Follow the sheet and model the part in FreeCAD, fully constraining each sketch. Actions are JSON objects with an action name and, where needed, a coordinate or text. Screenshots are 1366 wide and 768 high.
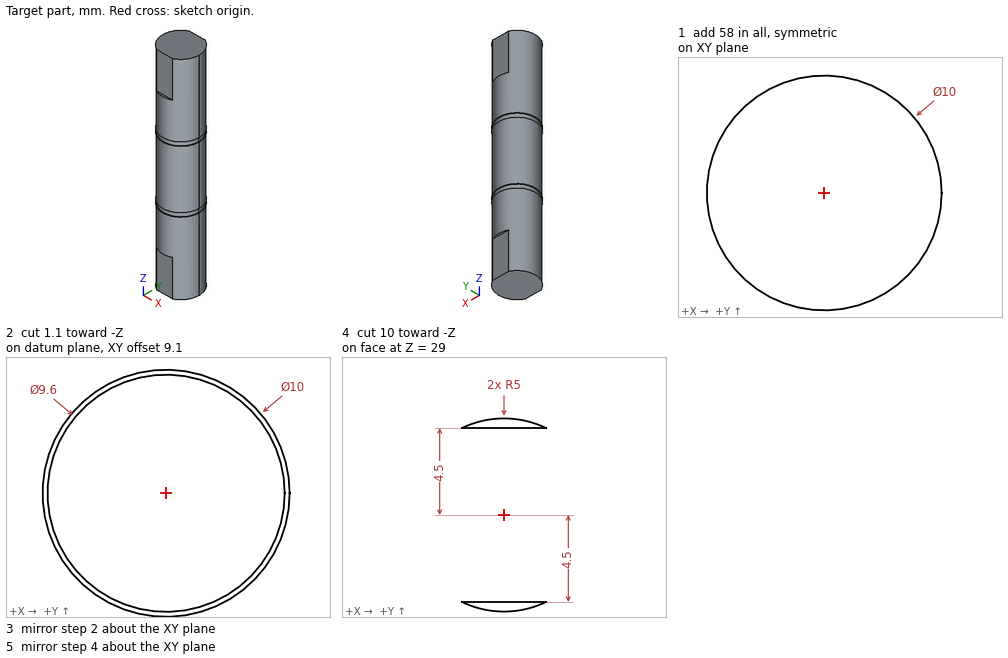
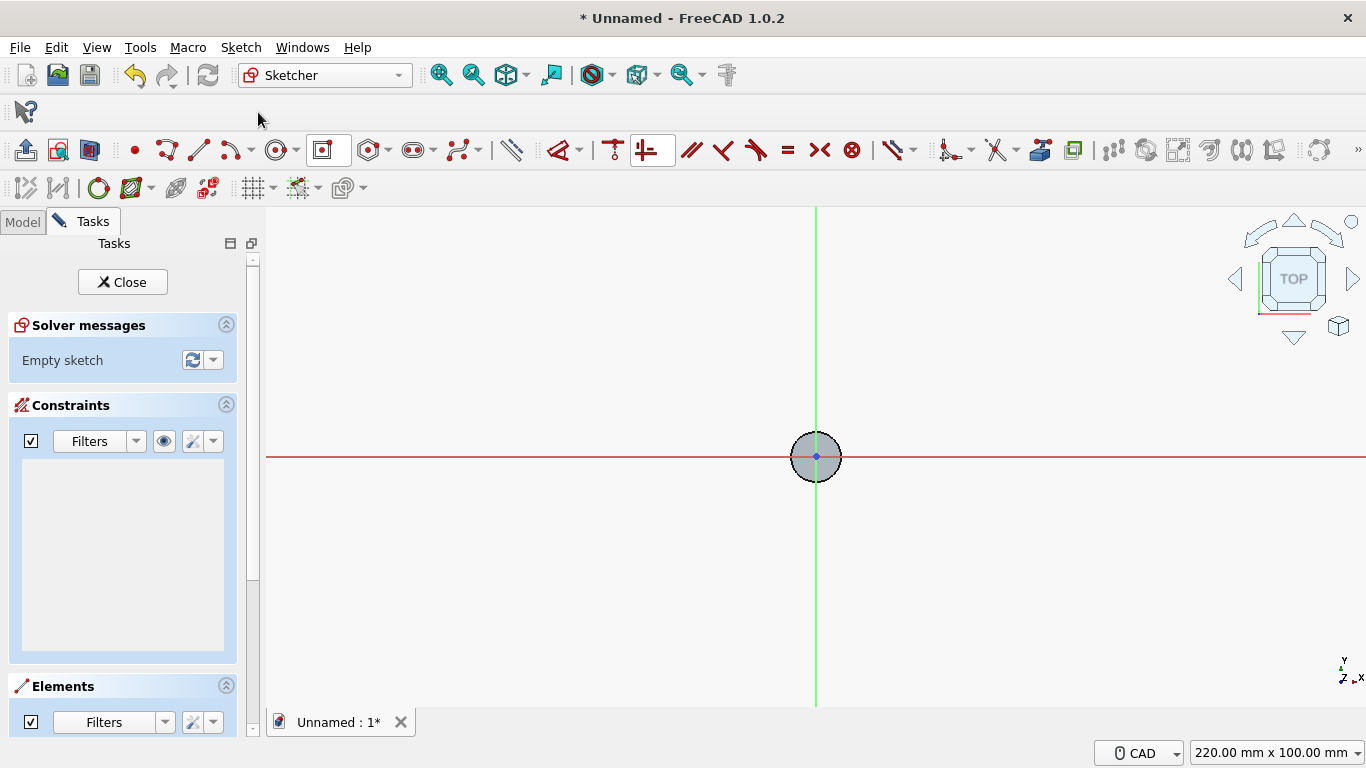
{"action": "scroll", "coordinate": [830, 457], "scroll_direction": "up", "scroll_amount": 9}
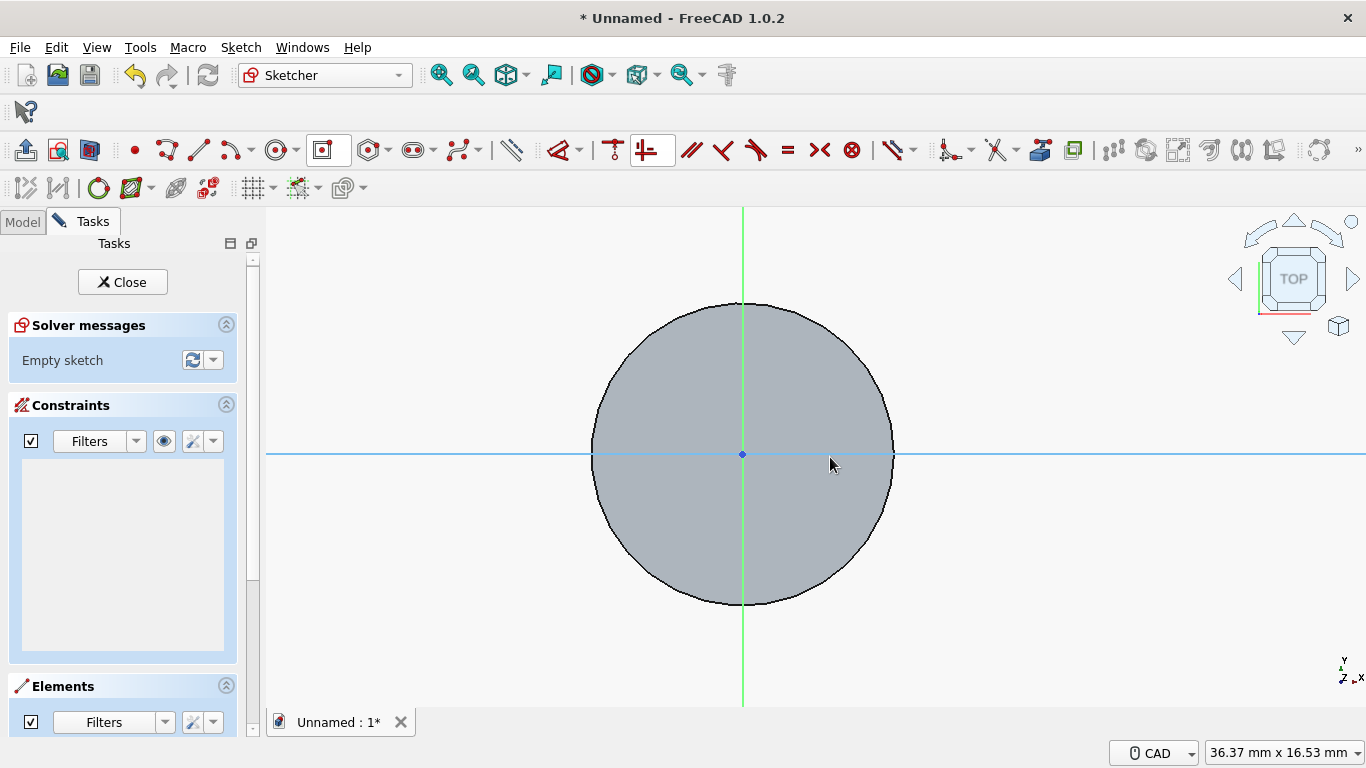
{"action": "left_click", "coordinate": [200, 150]}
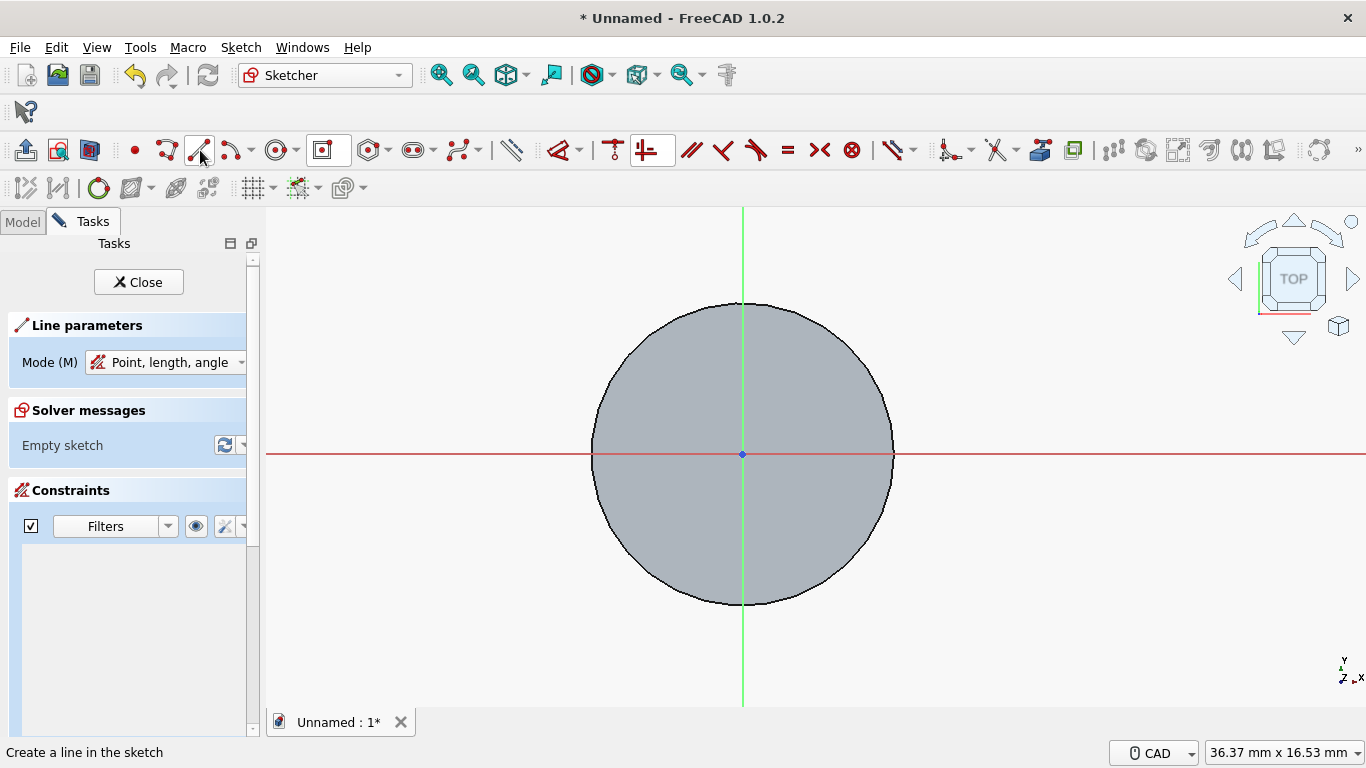
{"action": "left_click", "coordinate": [677, 318]}
{"action": "left_click", "coordinate": [809, 318]}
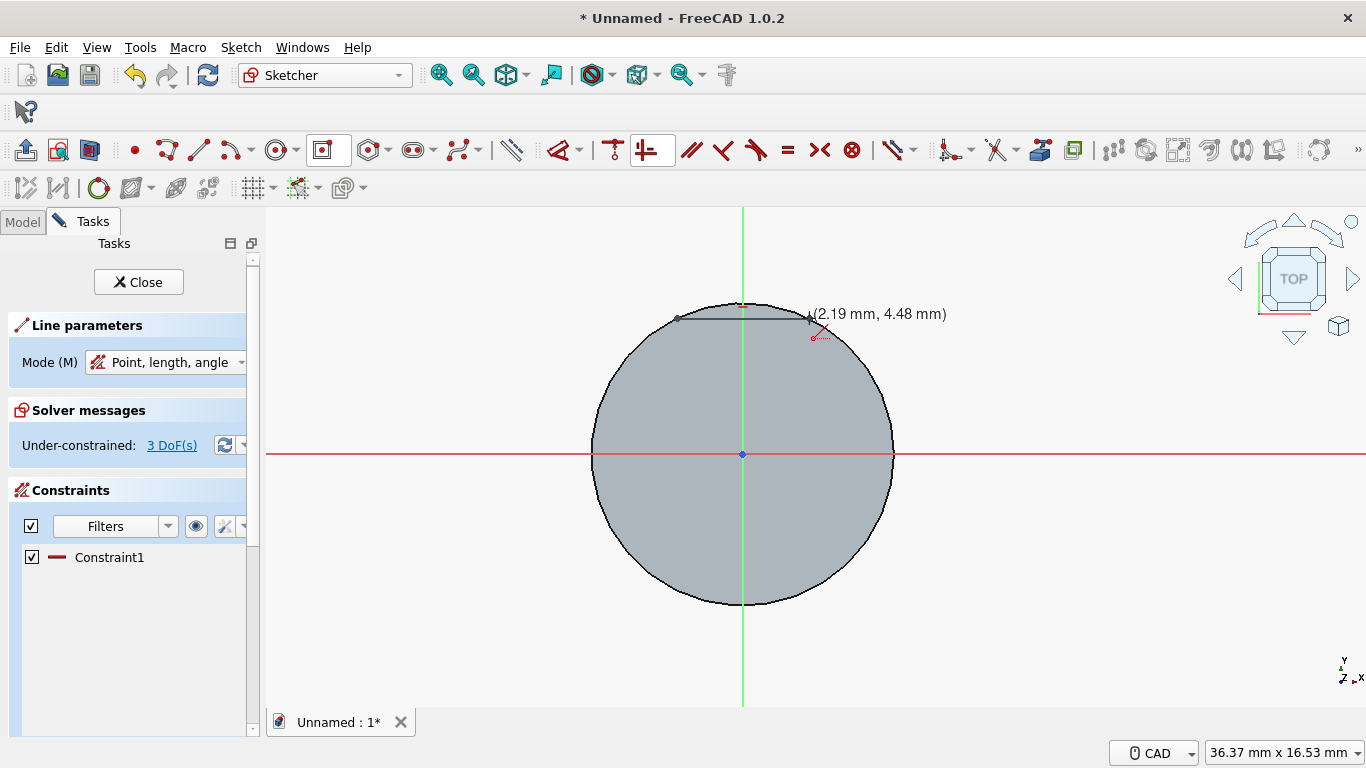
{"action": "left_click", "coordinate": [254, 150]}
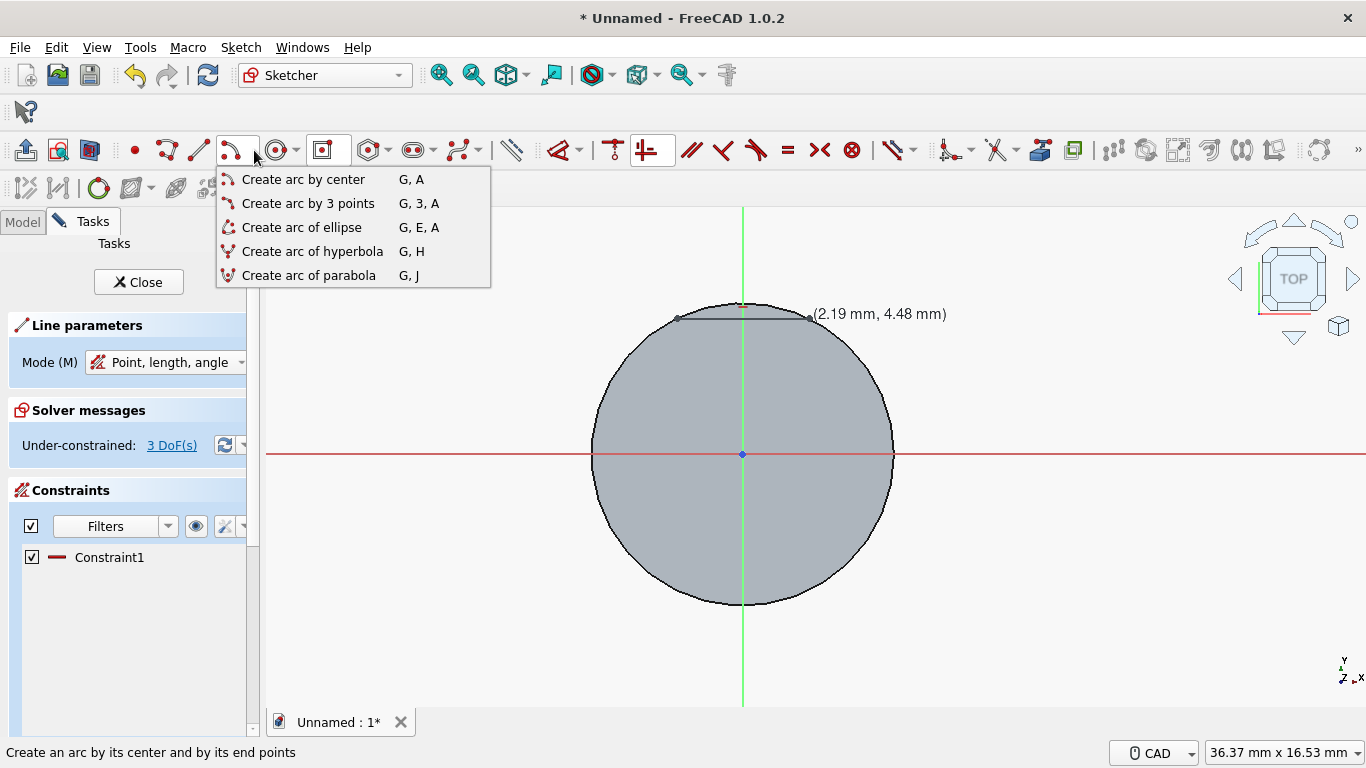
{"action": "left_click", "coordinate": [354, 203]}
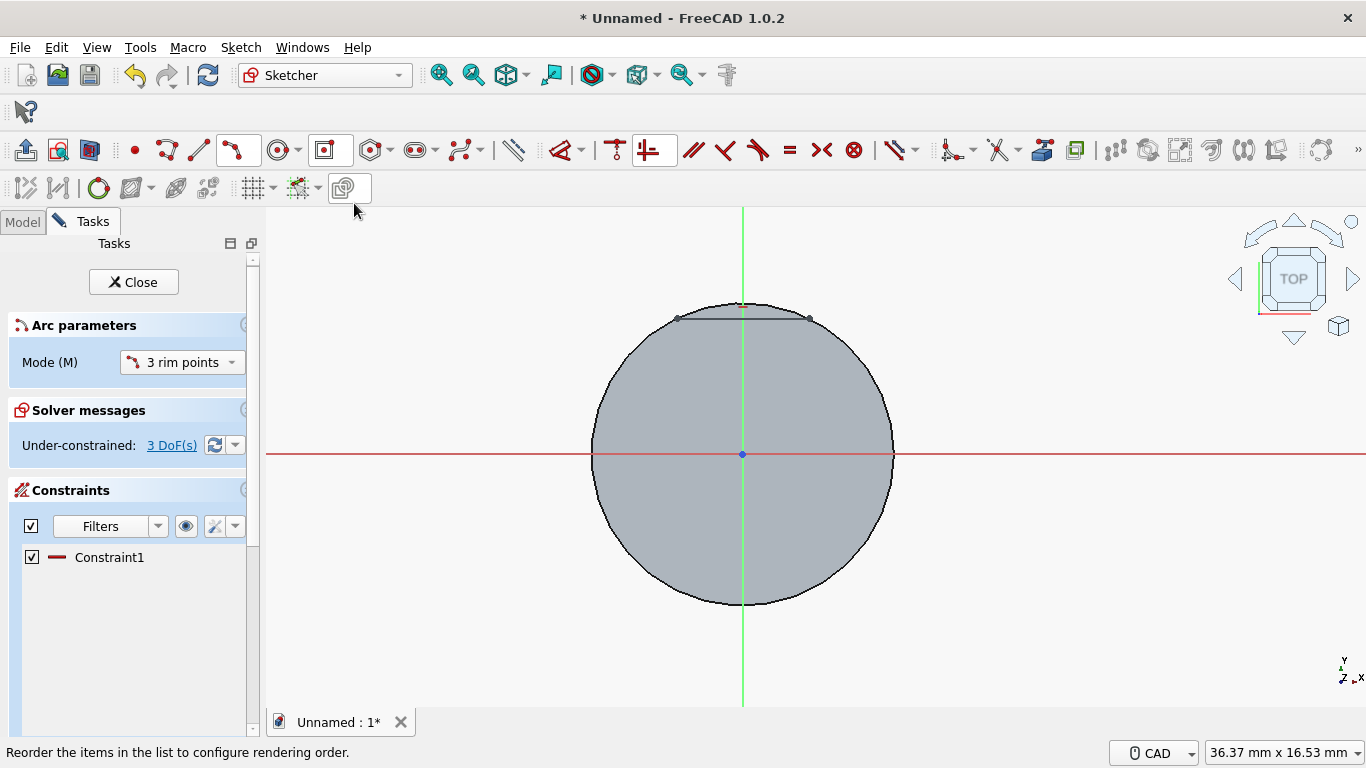
{"action": "left_click", "coordinate": [809, 319]}
{"action": "left_click", "coordinate": [677, 319]}
{"action": "left_click", "coordinate": [756, 304]}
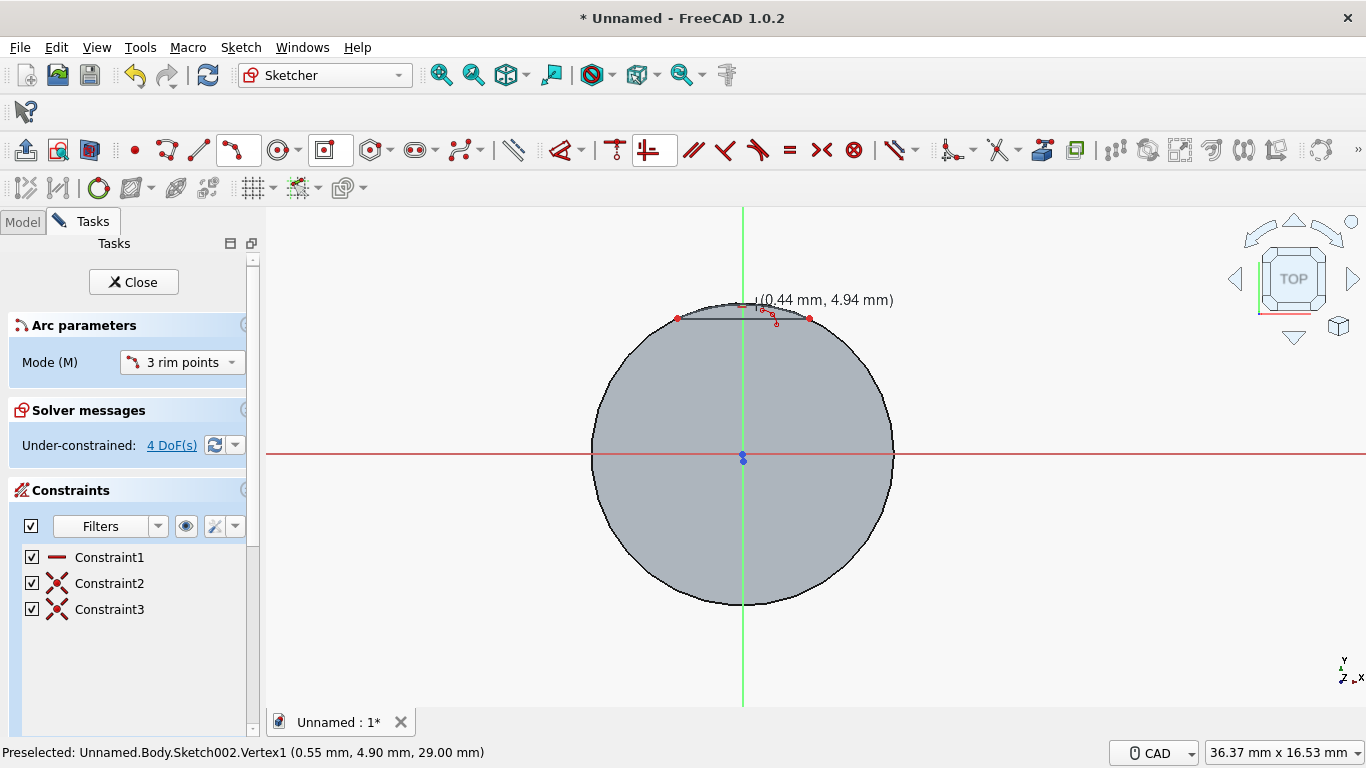
{"action": "key", "text": "g l"}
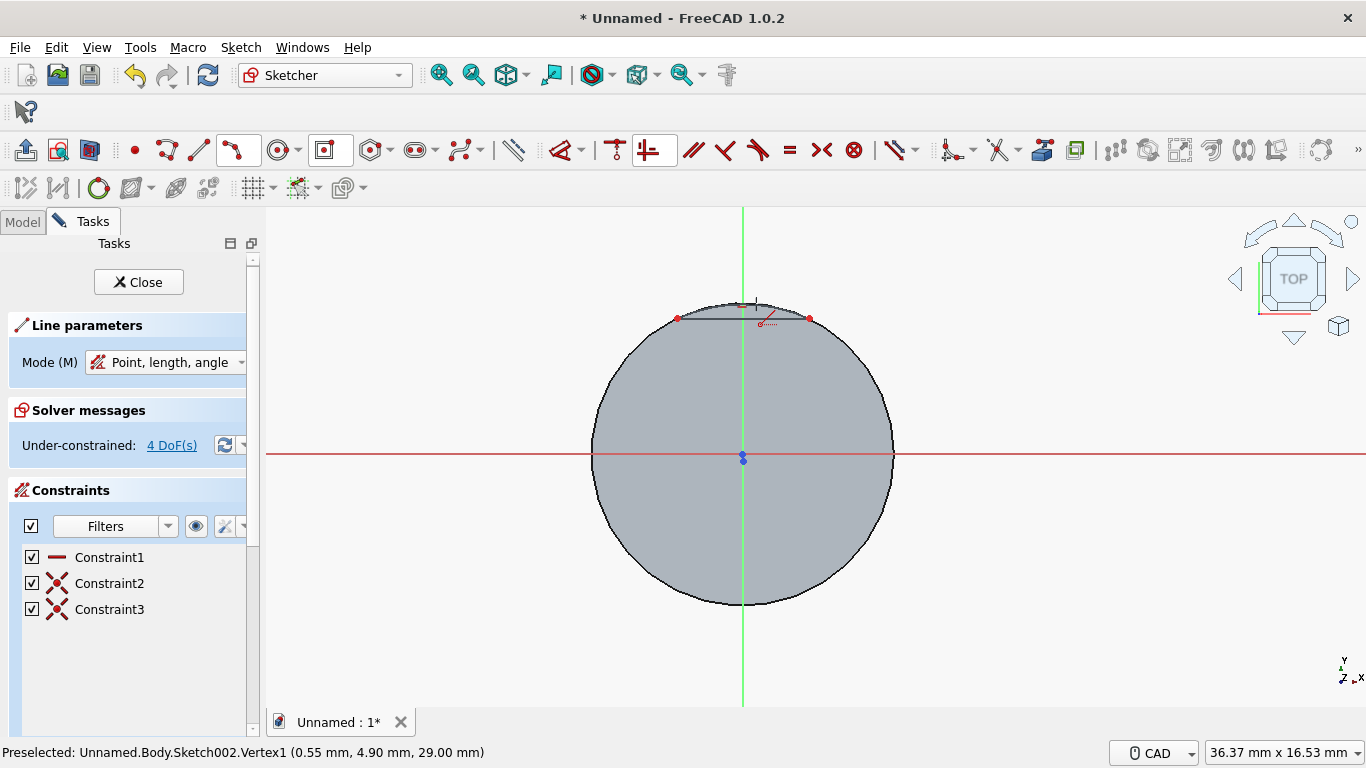
{"action": "left_click", "coordinate": [809, 591]}
{"action": "left_click", "coordinate": [677, 591]}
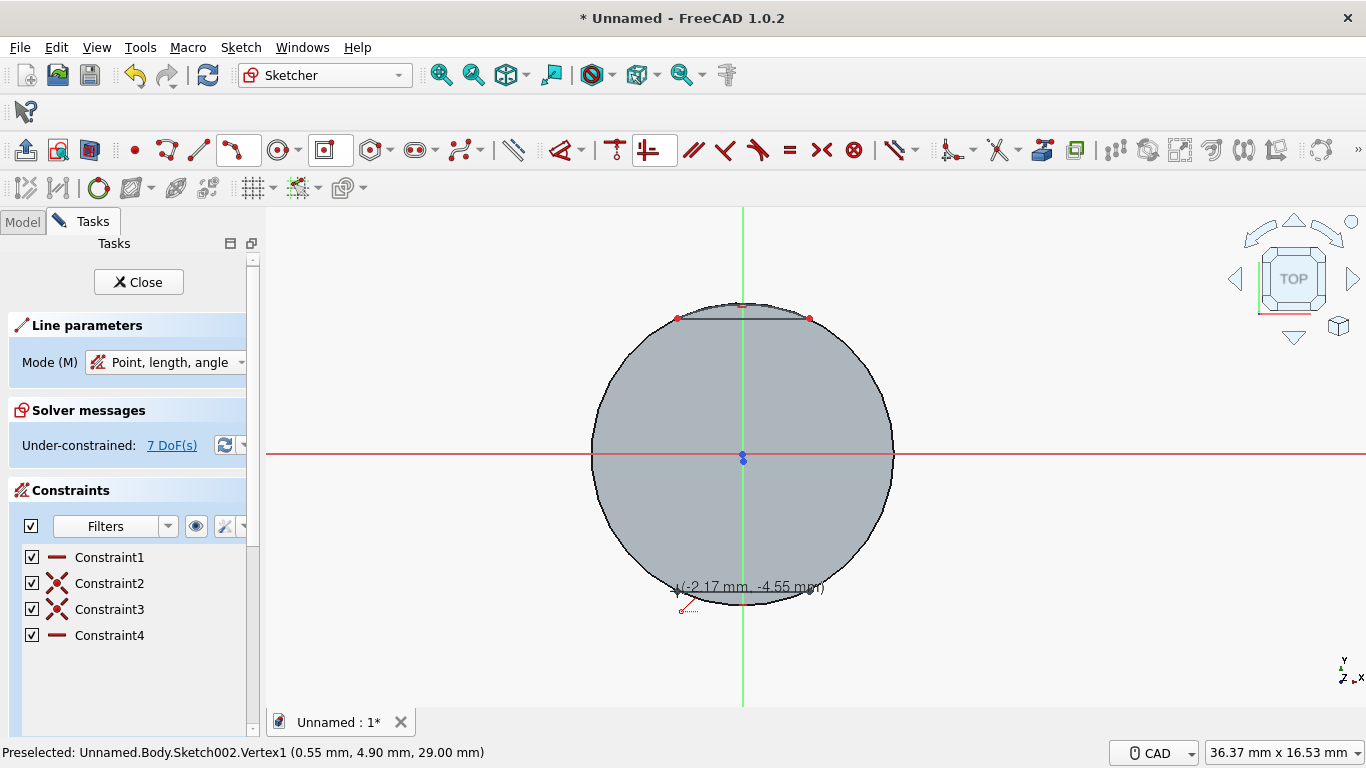
{"action": "left_click", "coordinate": [232, 150]}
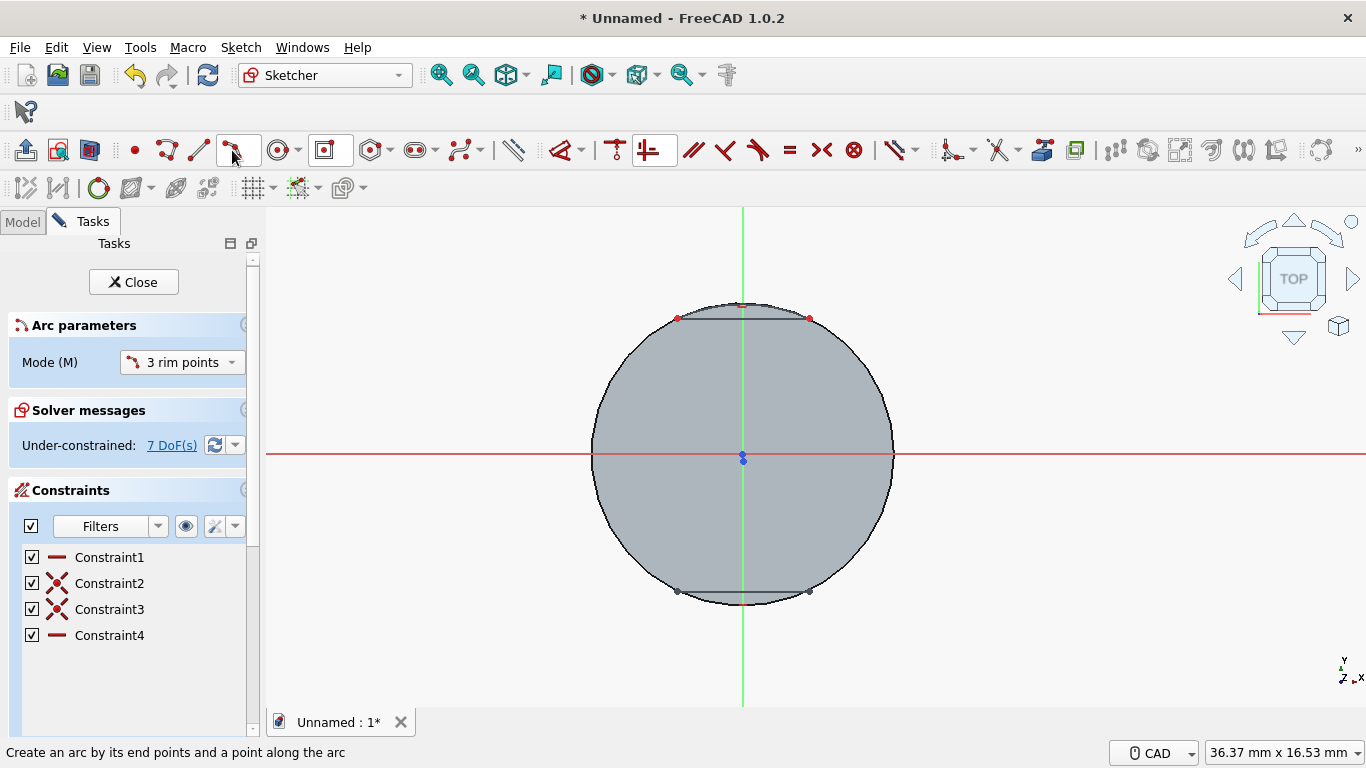
{"action": "left_click", "coordinate": [677, 592]}
{"action": "left_click", "coordinate": [809, 592]}
{"action": "left_click", "coordinate": [756, 605]}
{"action": "key", "text": "Escape"}